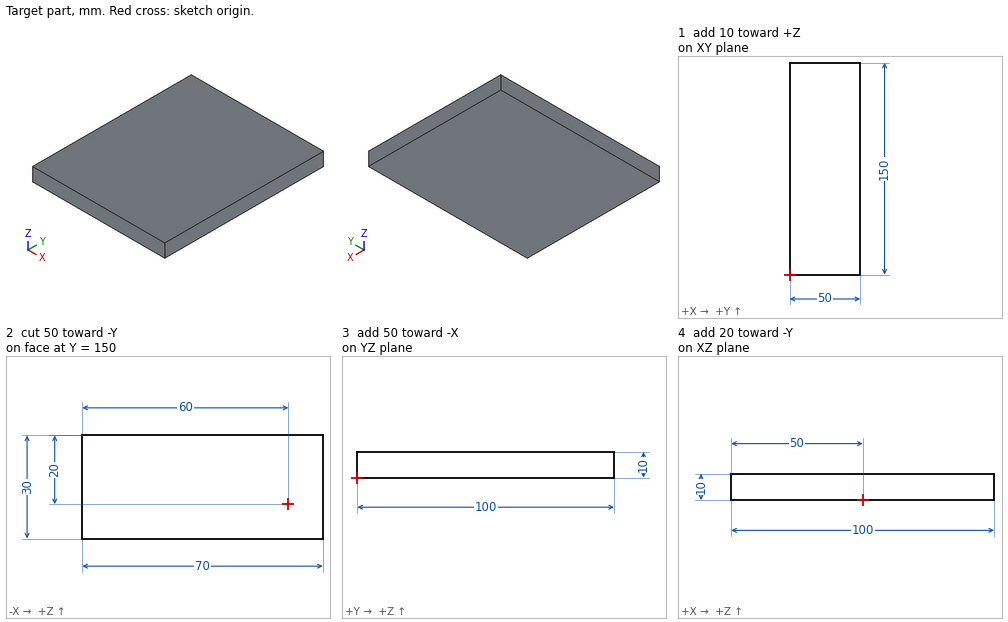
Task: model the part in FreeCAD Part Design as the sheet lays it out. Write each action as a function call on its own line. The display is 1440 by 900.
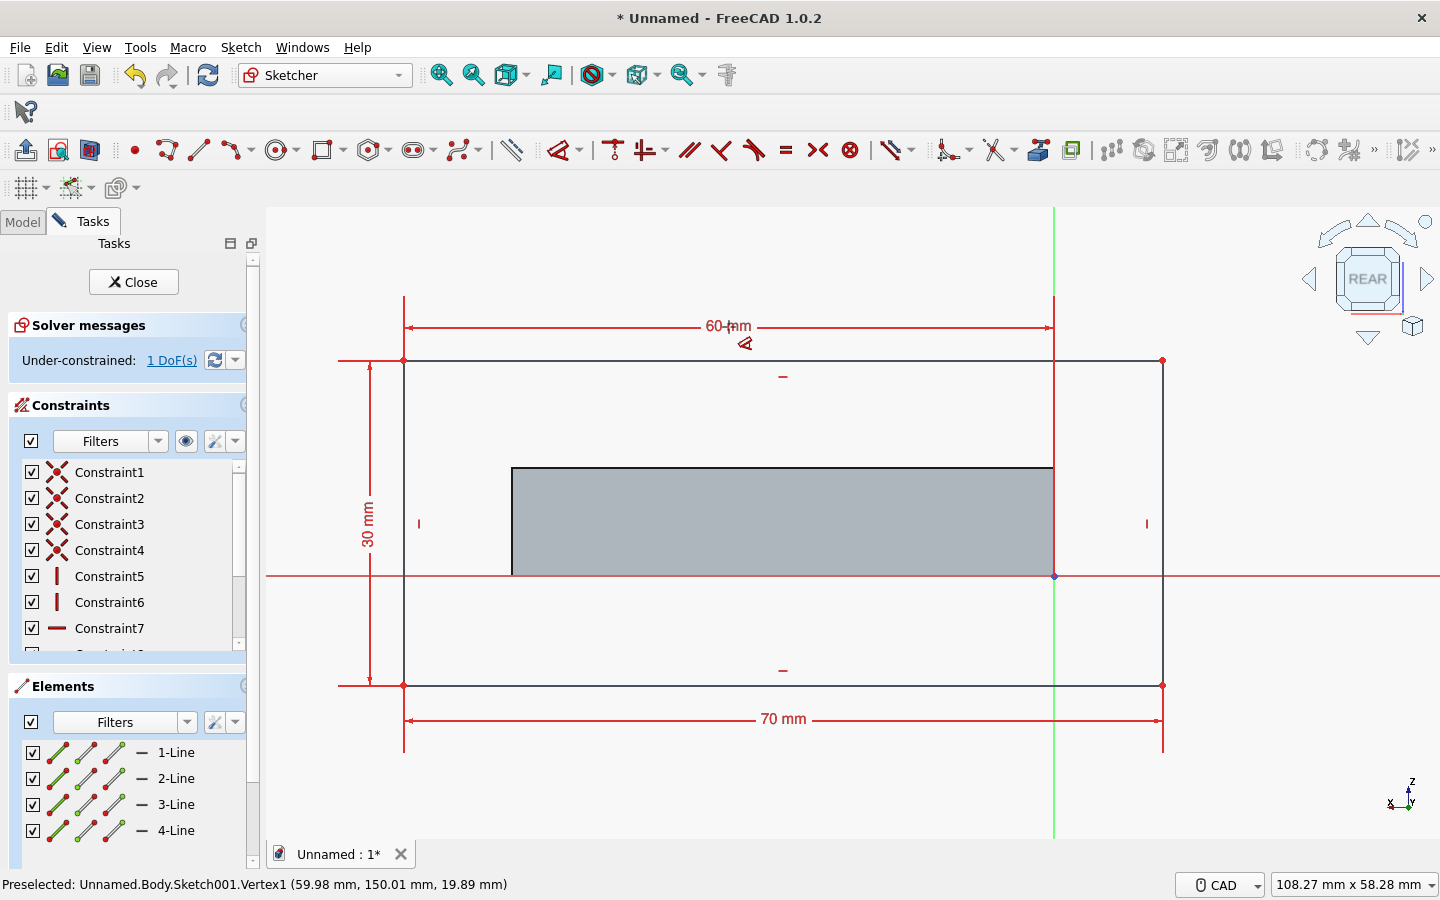
click(404, 361)
click(370, 469)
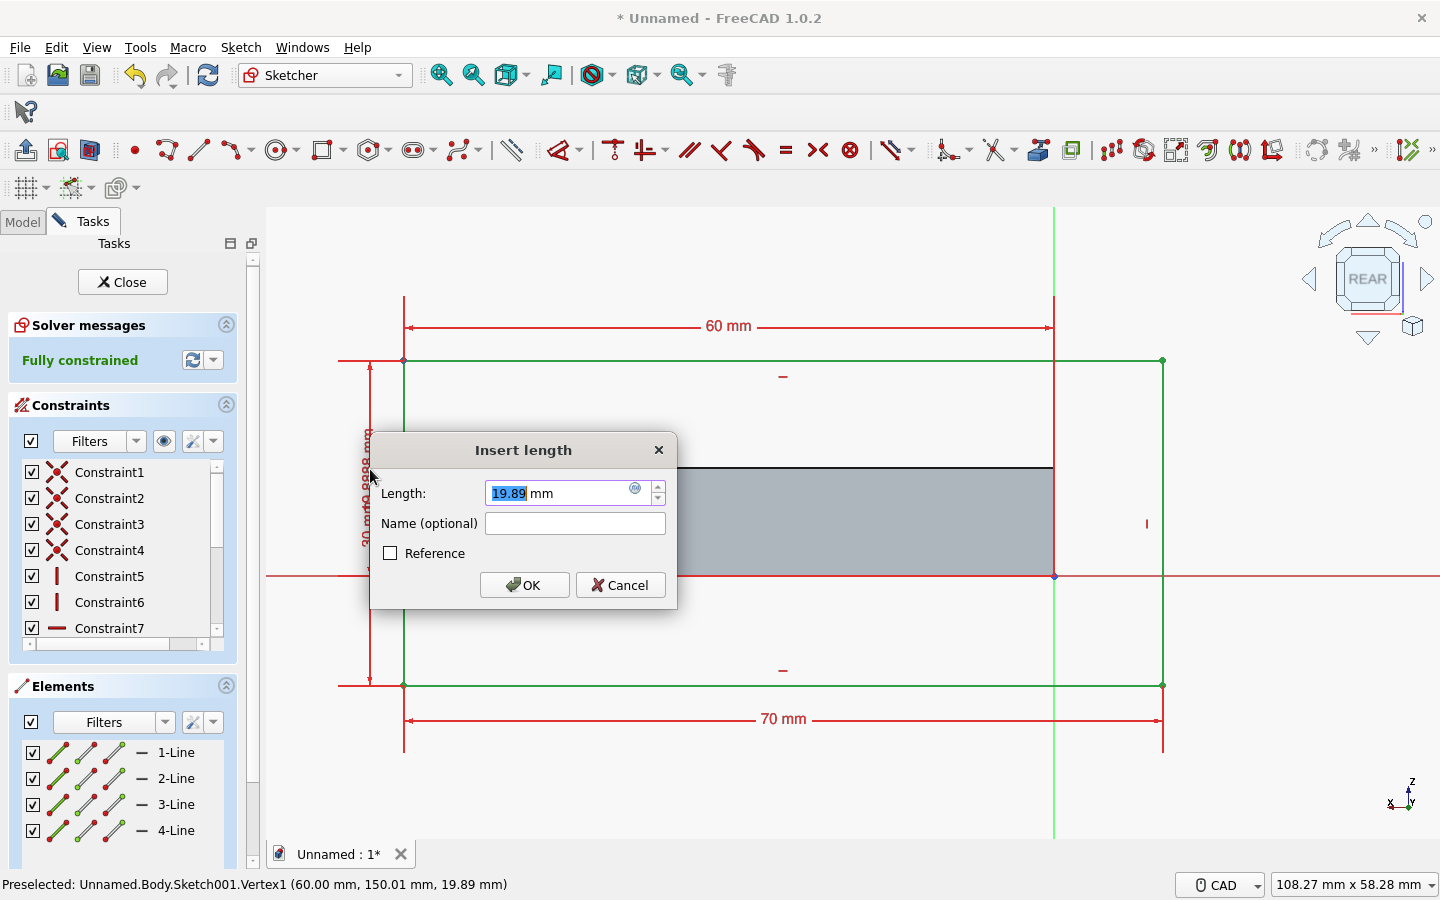
text(20)
key(Return)
key(Escape)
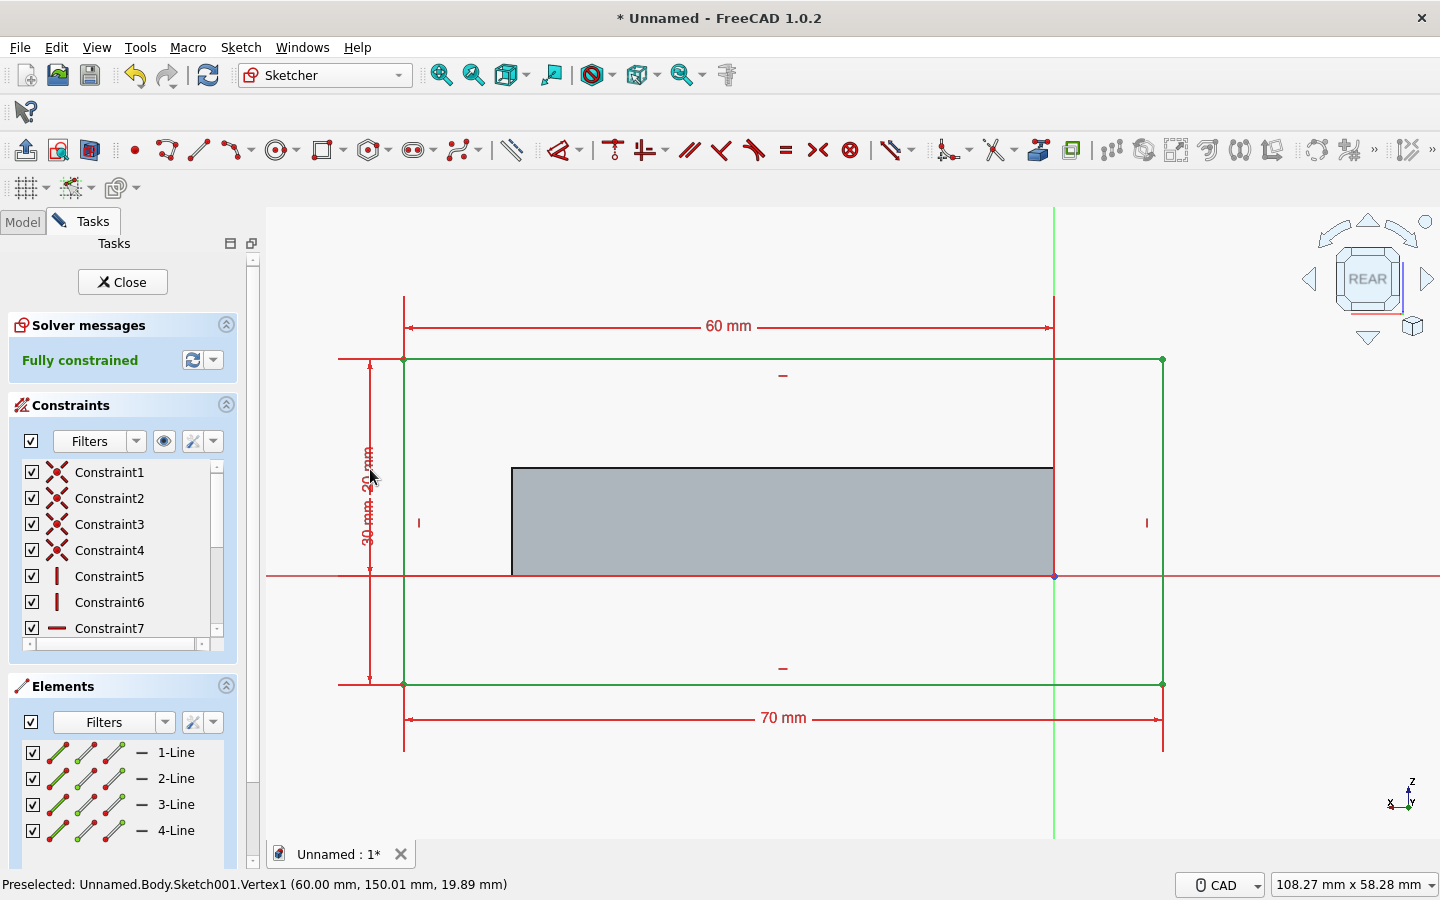
click(123, 282)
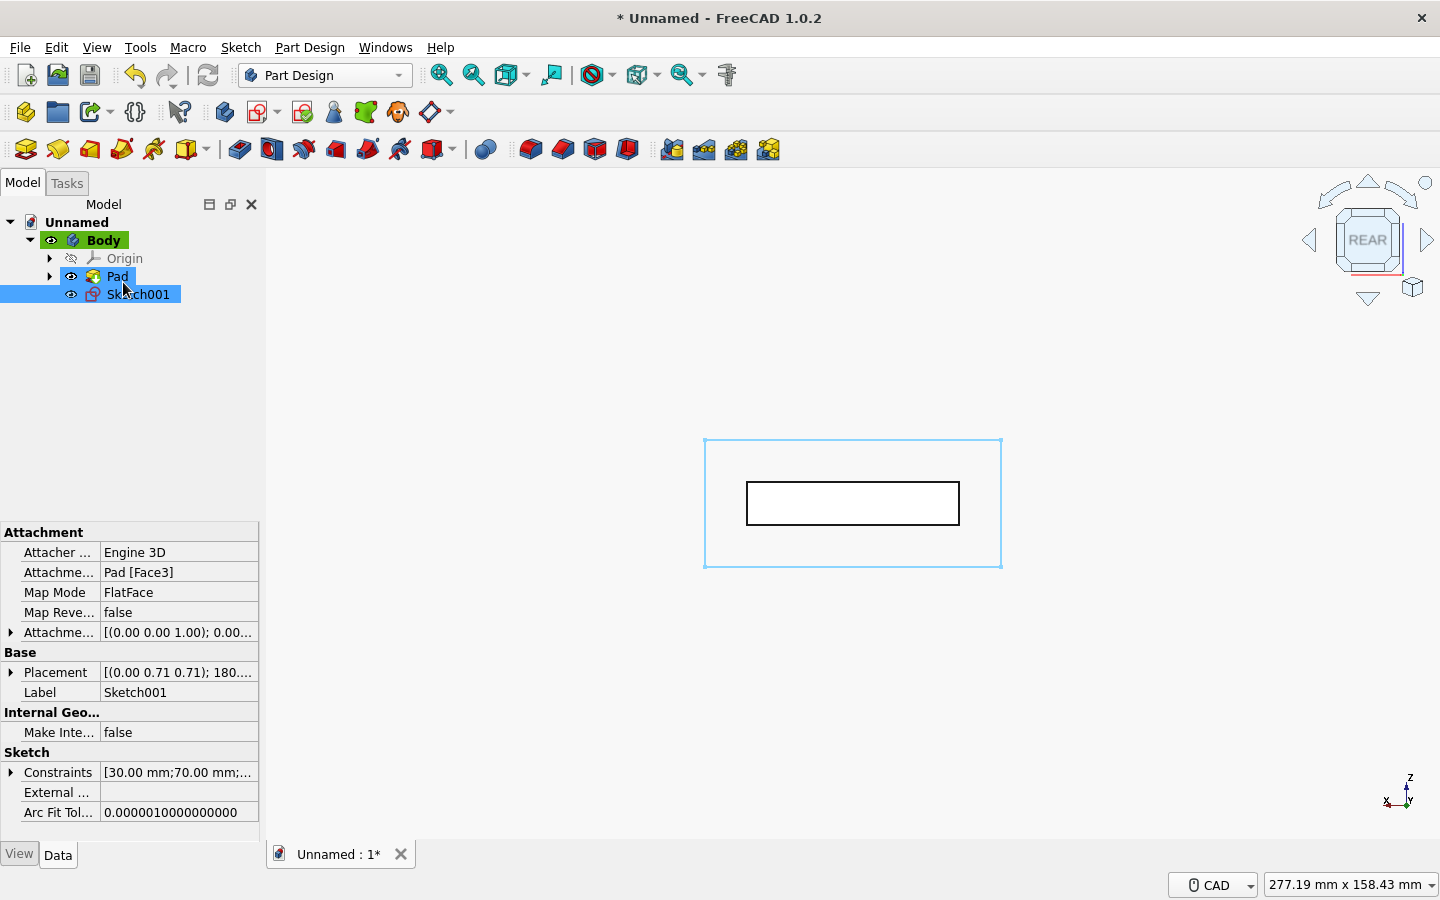
click(240, 150)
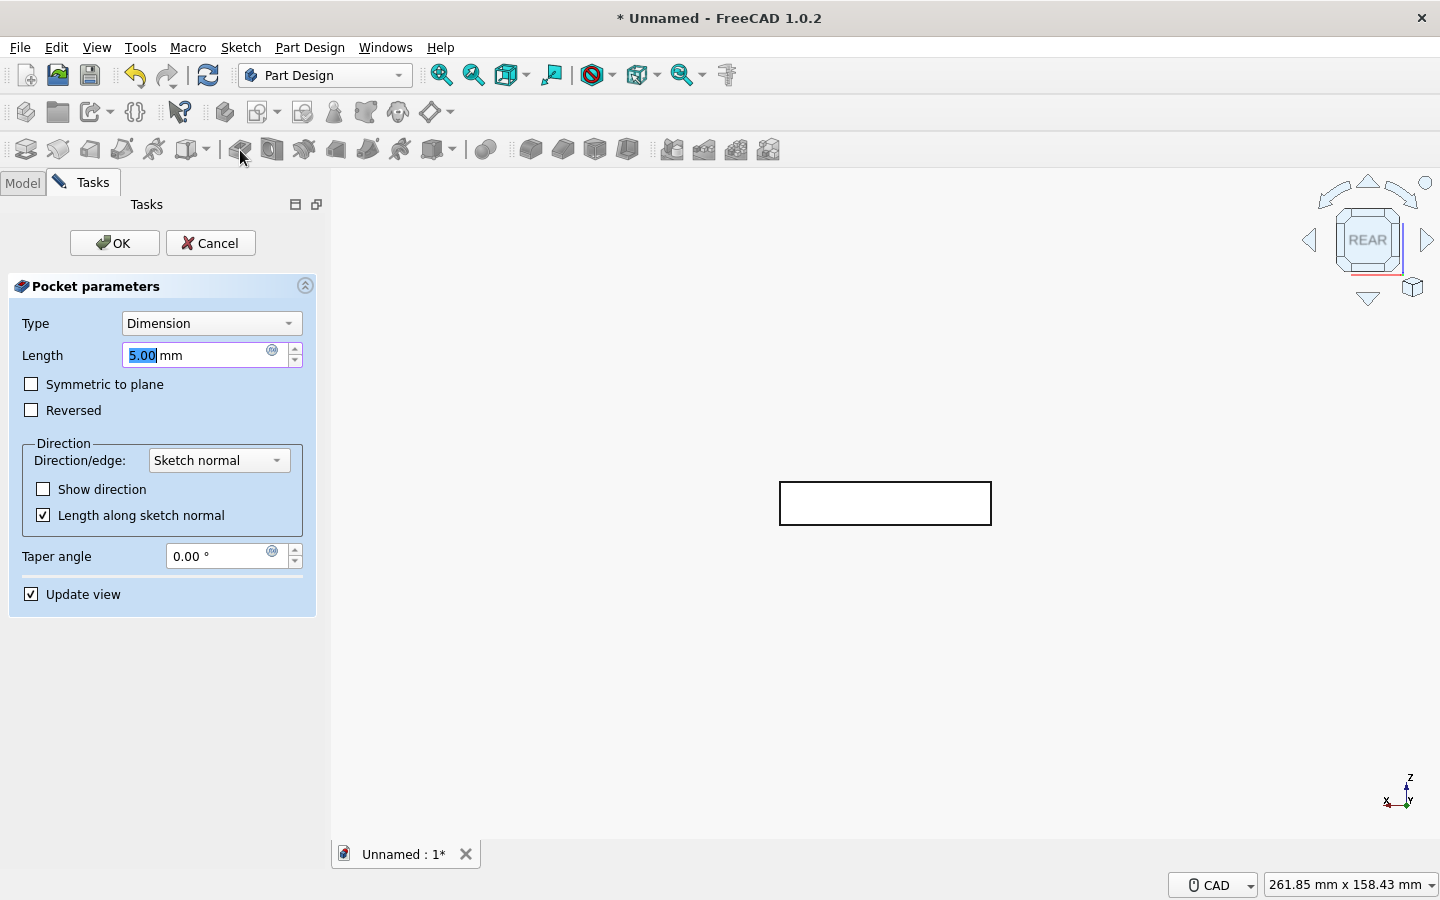
text(50)
key(Tab)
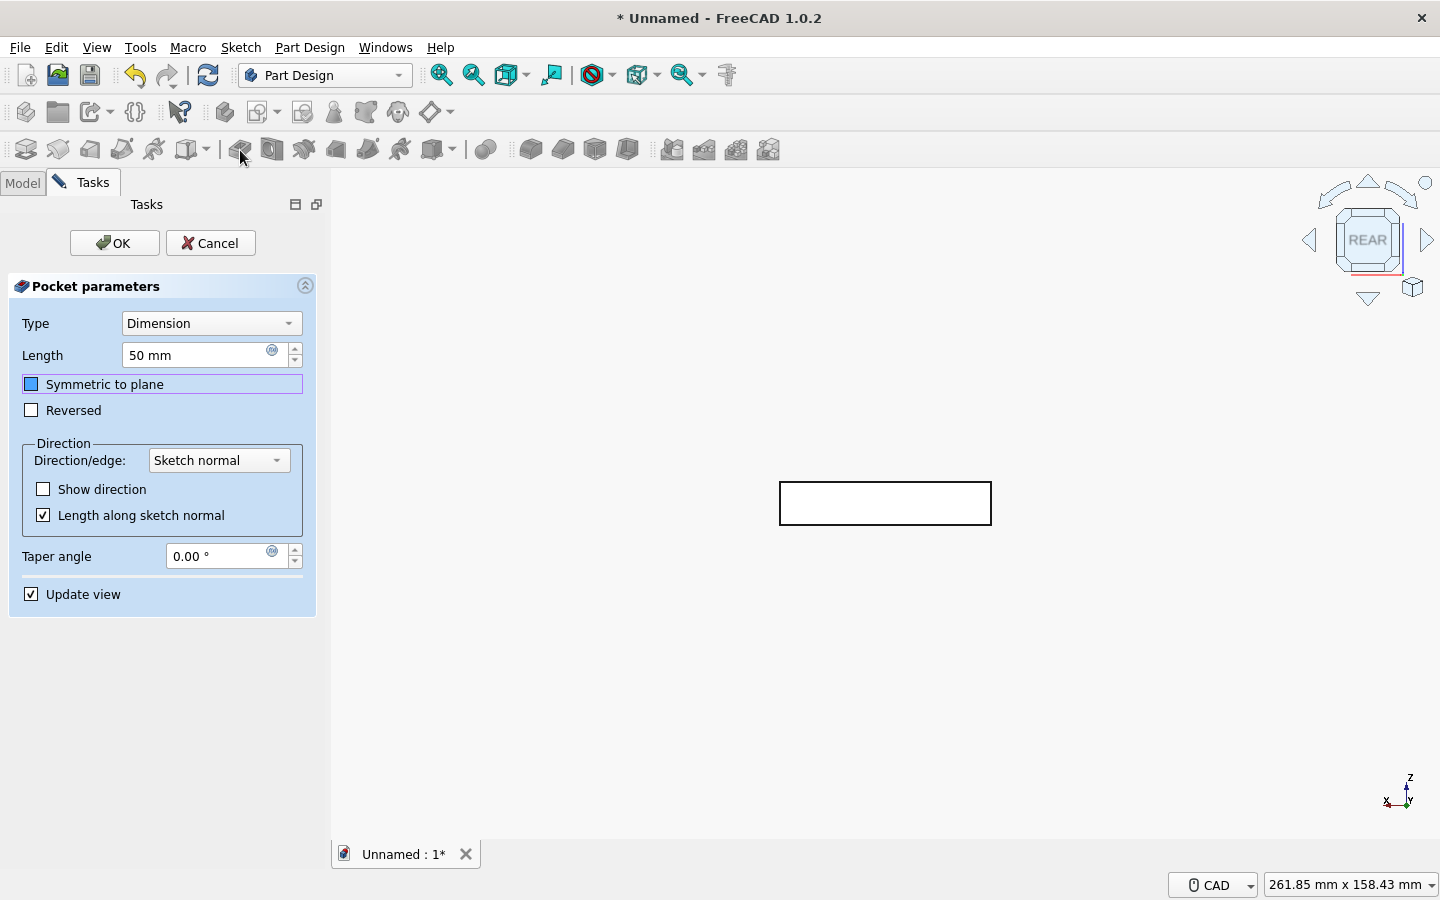
click(115, 243)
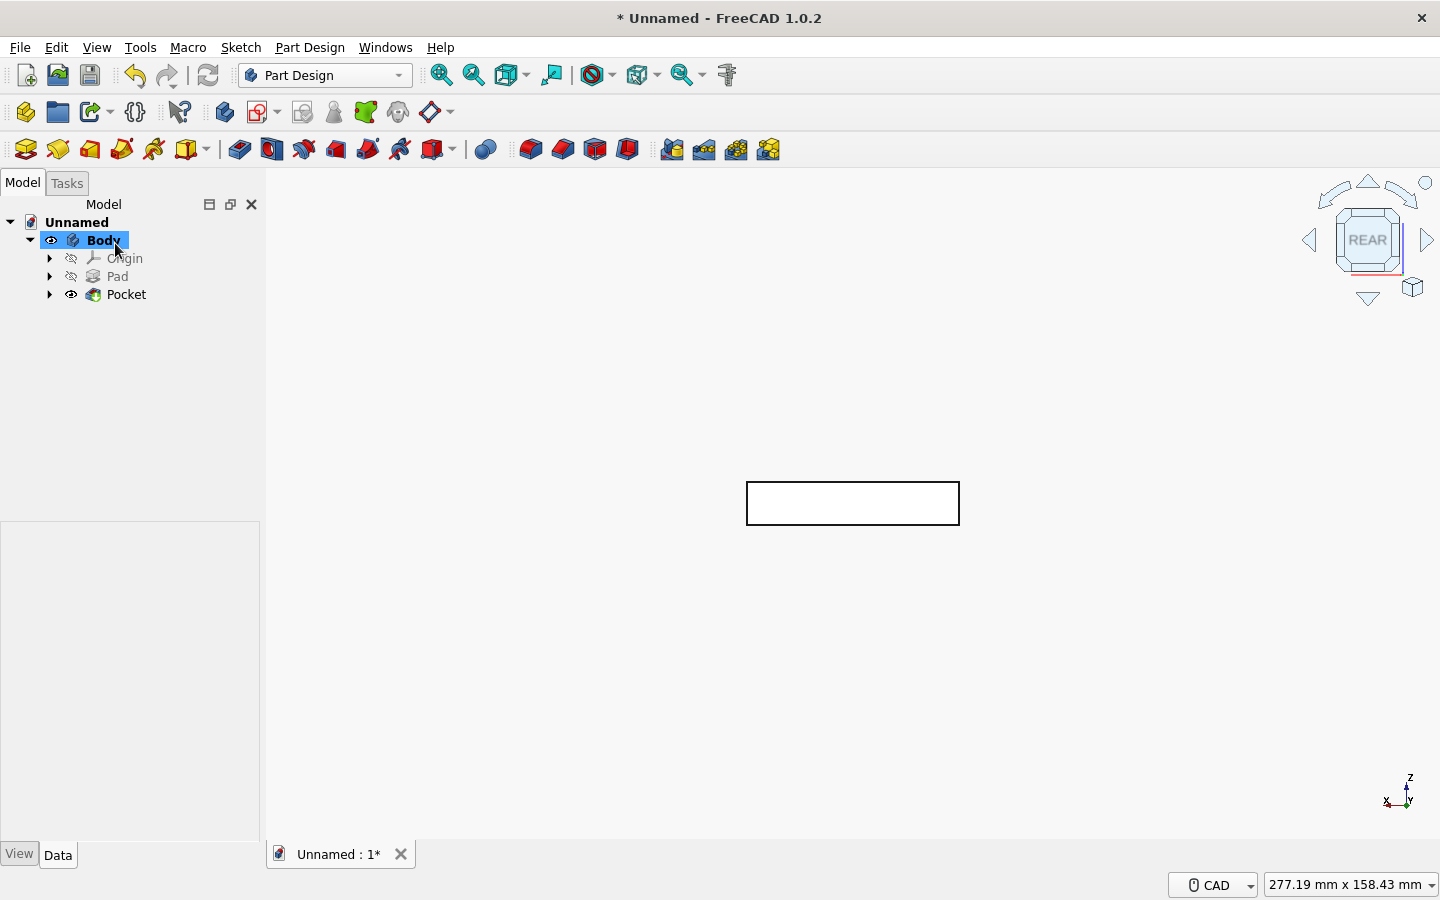
click(442, 76)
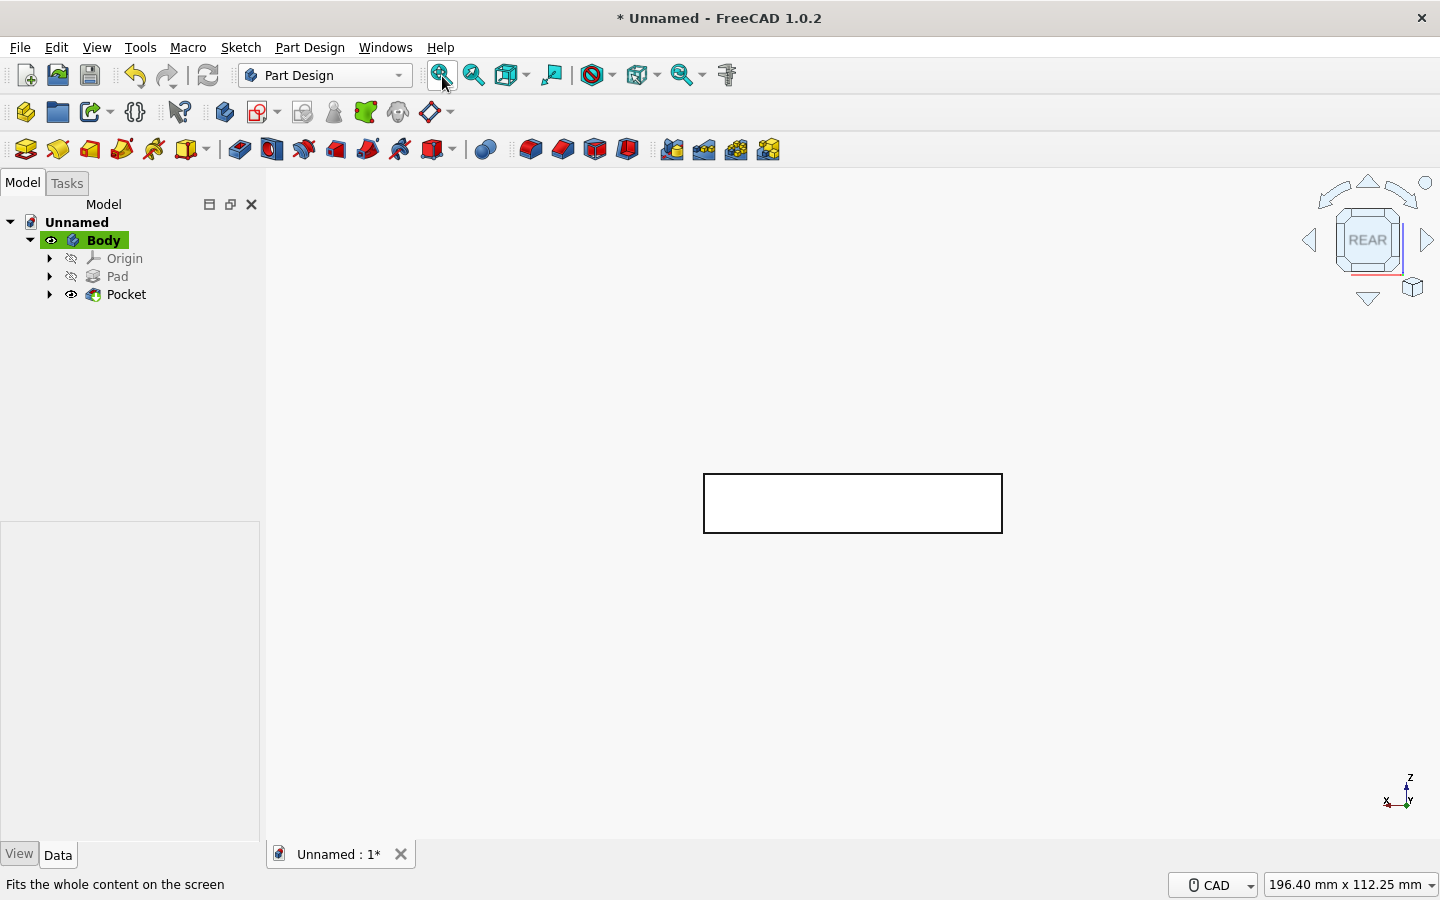
click(258, 112)